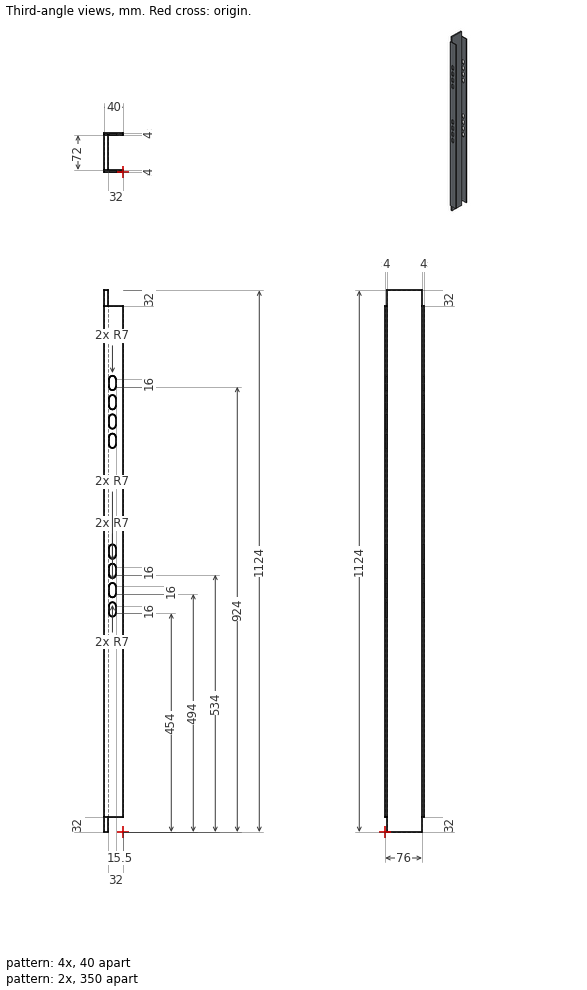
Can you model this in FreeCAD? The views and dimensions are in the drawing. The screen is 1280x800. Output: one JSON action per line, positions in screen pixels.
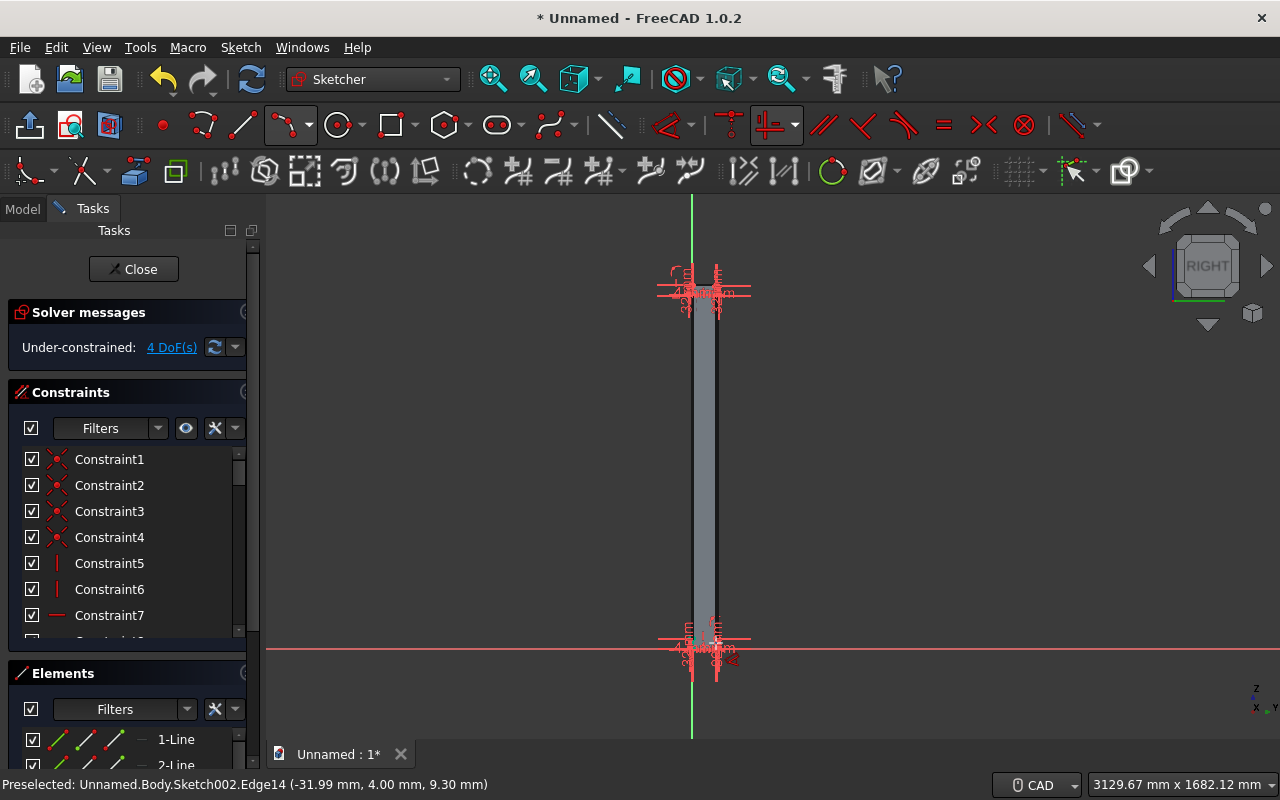
{"action": "scroll", "coordinate": [716, 286], "scroll_direction": "up", "scroll_amount": 12}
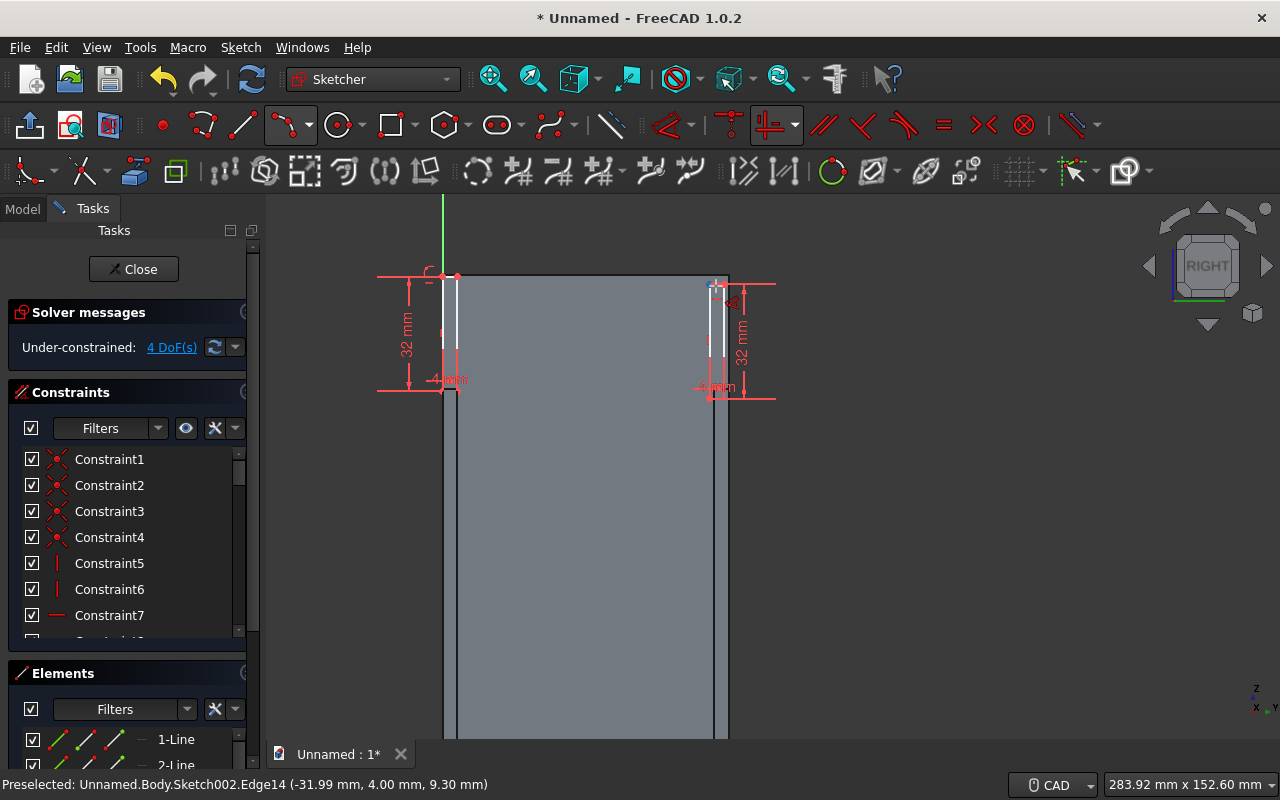
{"action": "left_click", "coordinate": [710, 284]}
{"action": "left_click", "coordinate": [576, 250]}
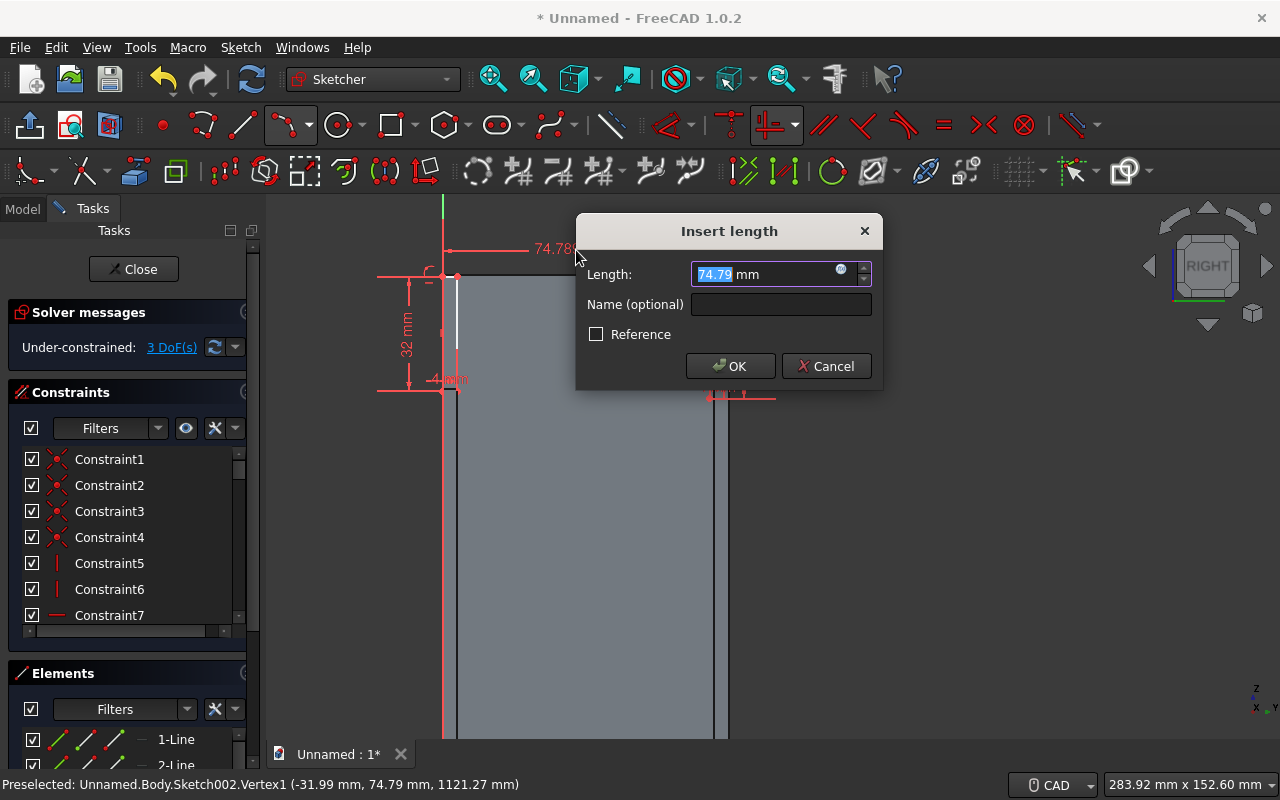
{"action": "type", "text": "76"}
{"action": "key", "text": "Return"}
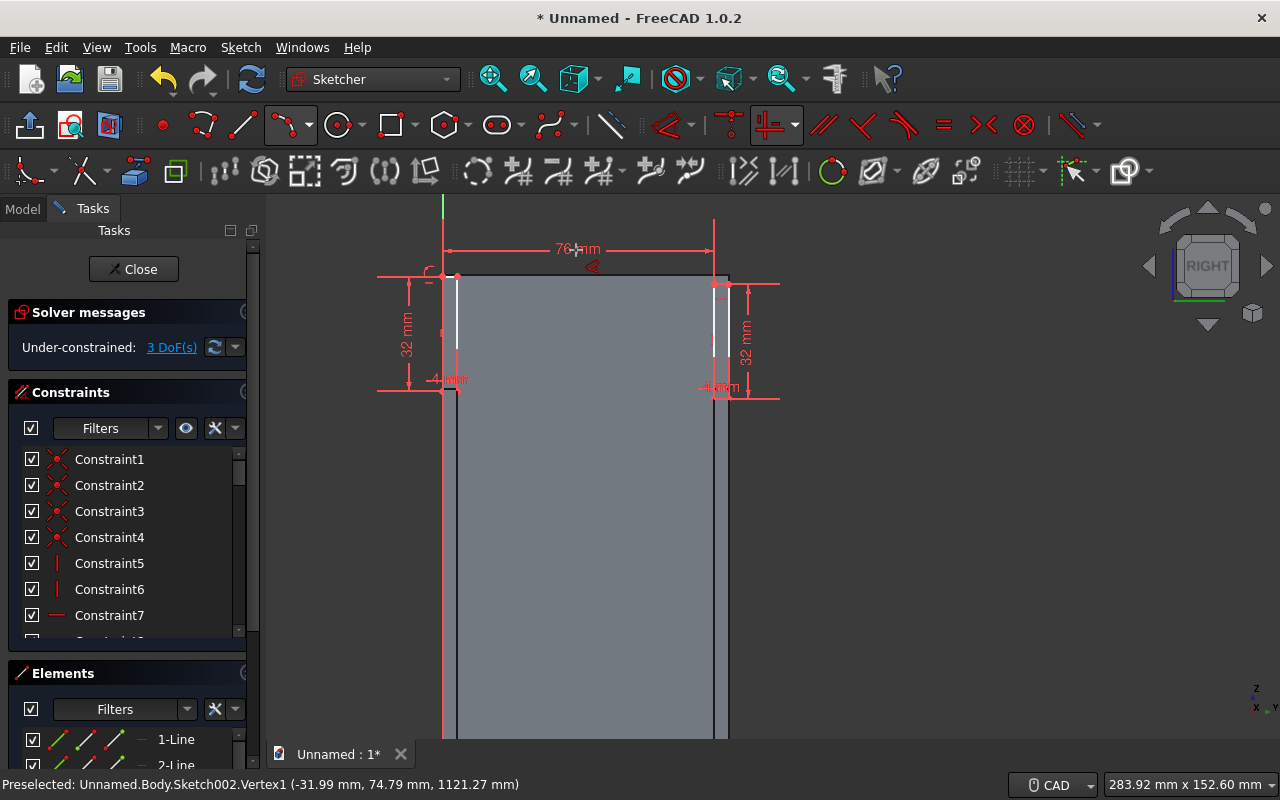
{"action": "scroll", "coordinate": [716, 285], "scroll_direction": "down", "scroll_amount": 12}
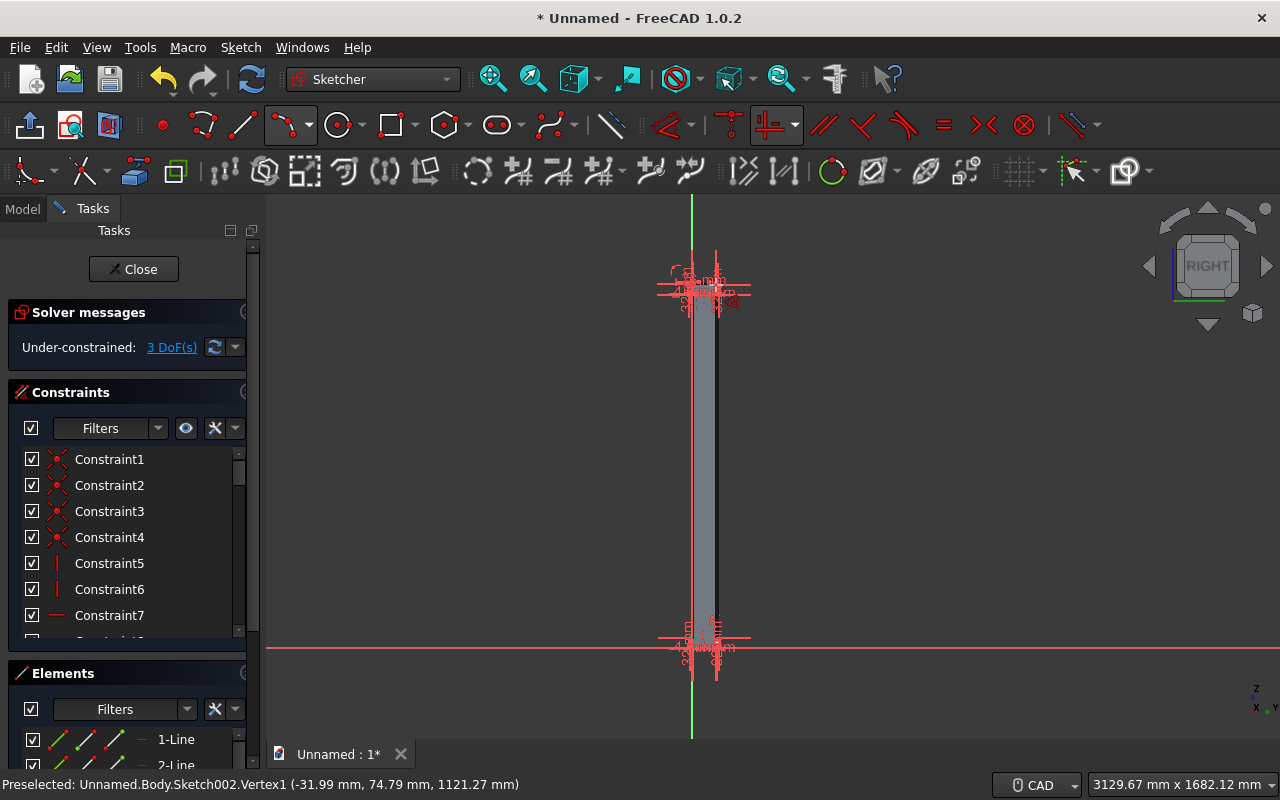
{"action": "scroll", "coordinate": [716, 638], "scroll_direction": "up", "scroll_amount": 12}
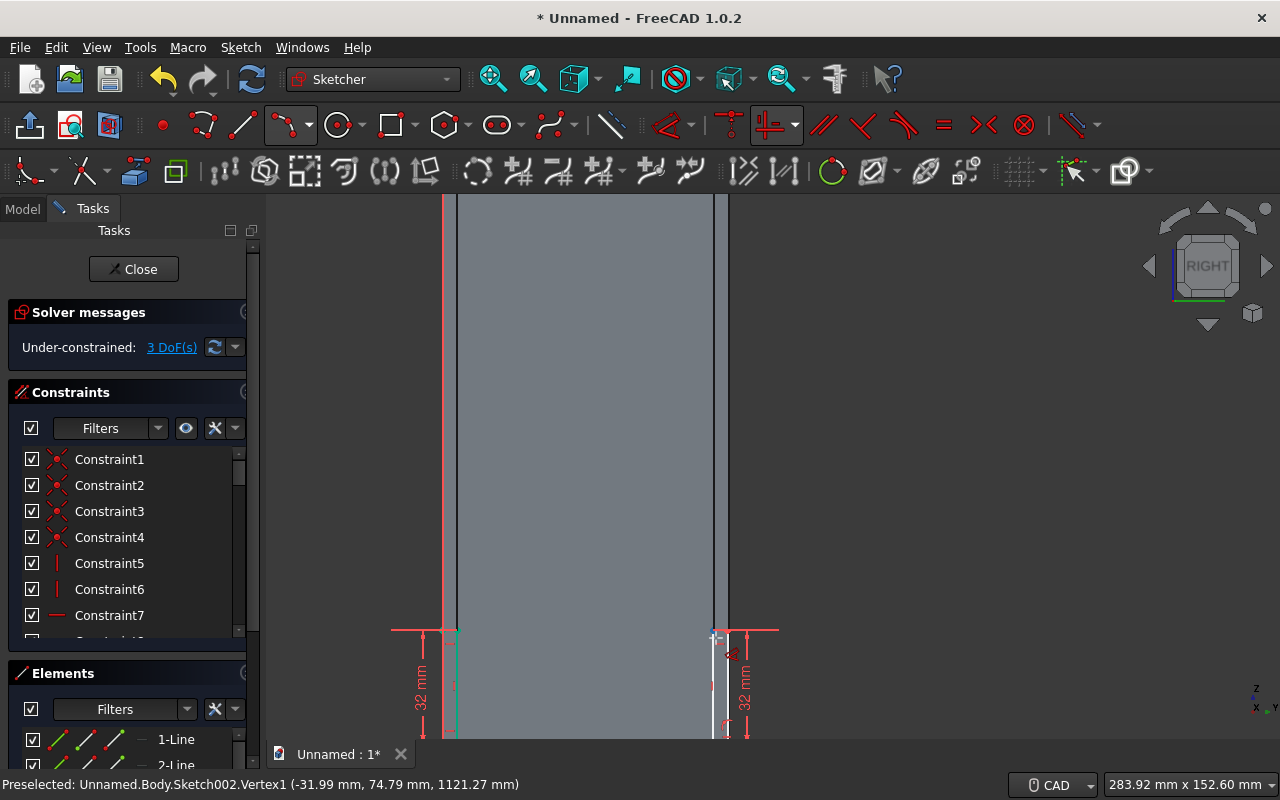
{"action": "left_click", "coordinate": [713, 630]}
{"action": "left_click", "coordinate": [578, 596]}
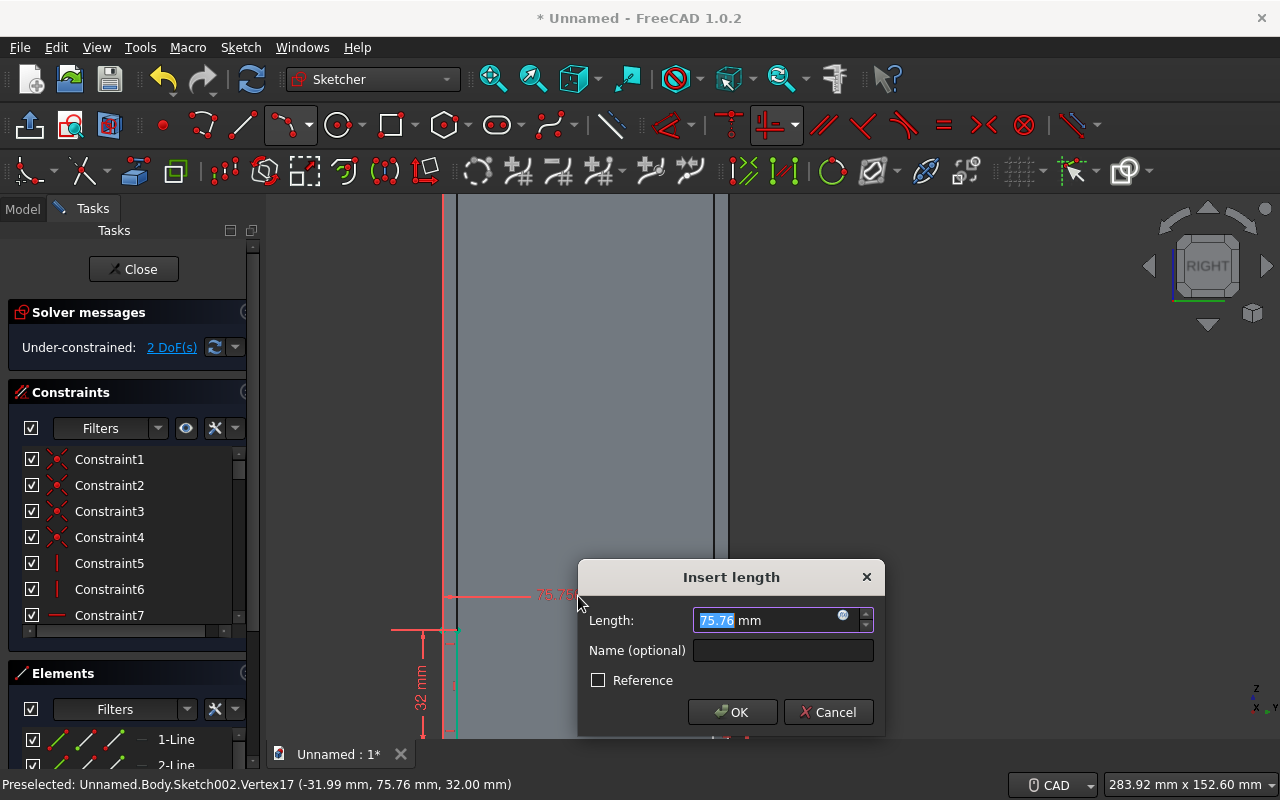
{"action": "type", "text": "76"}
{"action": "key", "text": "Return"}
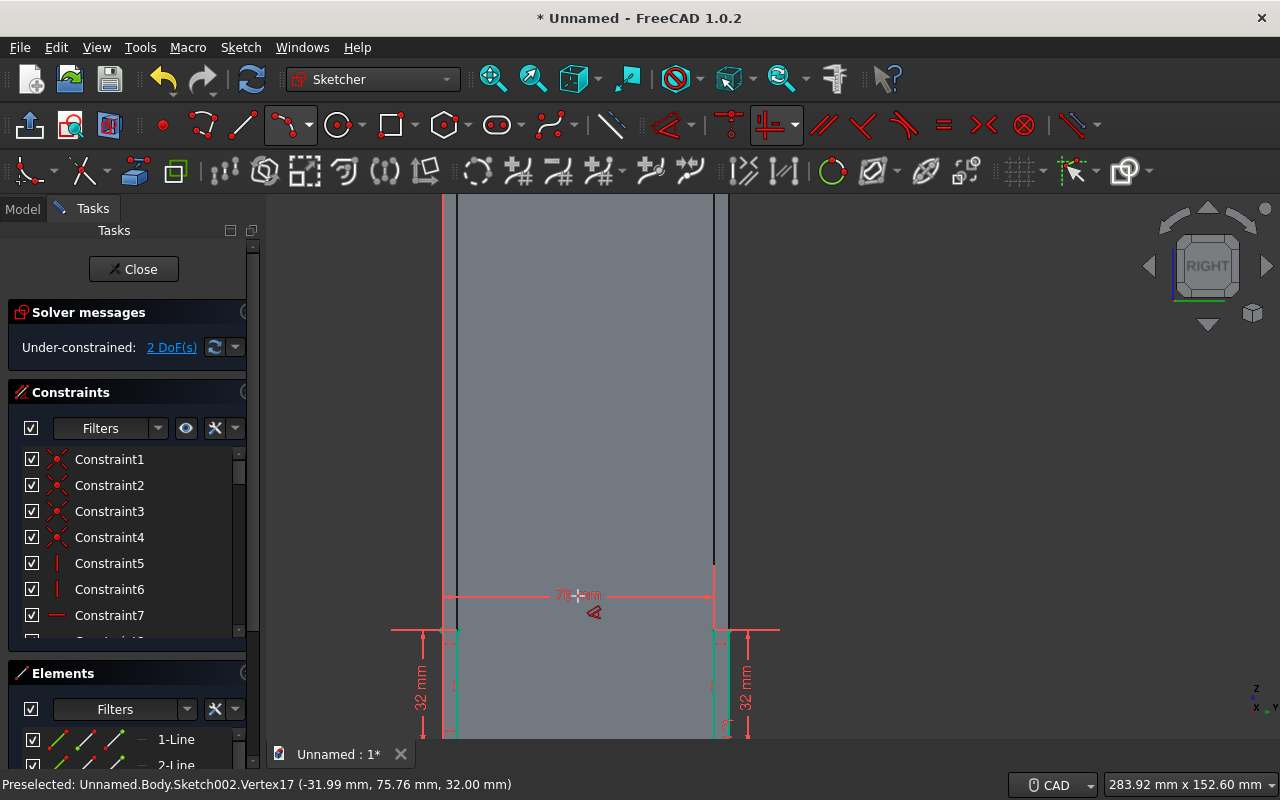
{"action": "scroll", "coordinate": [716, 639], "scroll_direction": "down", "scroll_amount": 12}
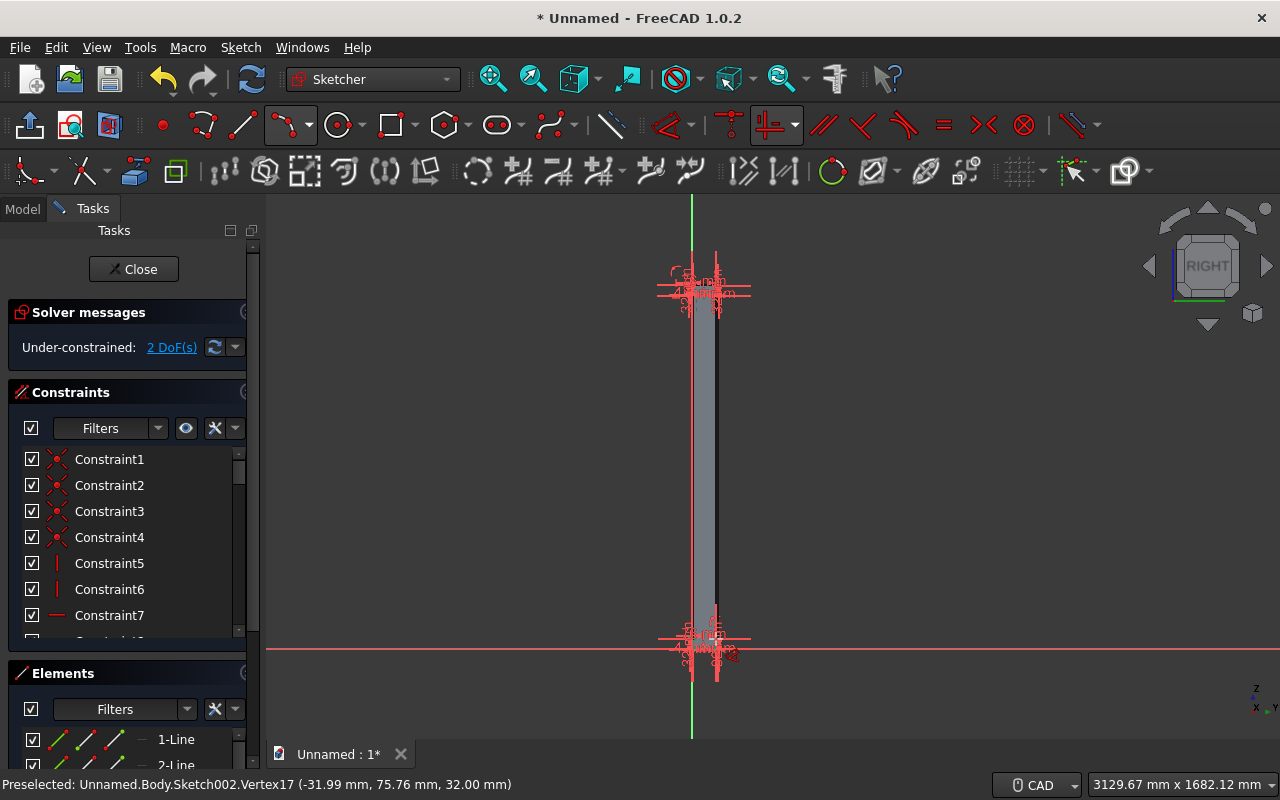
{"action": "scroll", "coordinate": [716, 286], "scroll_direction": "up", "scroll_amount": 12}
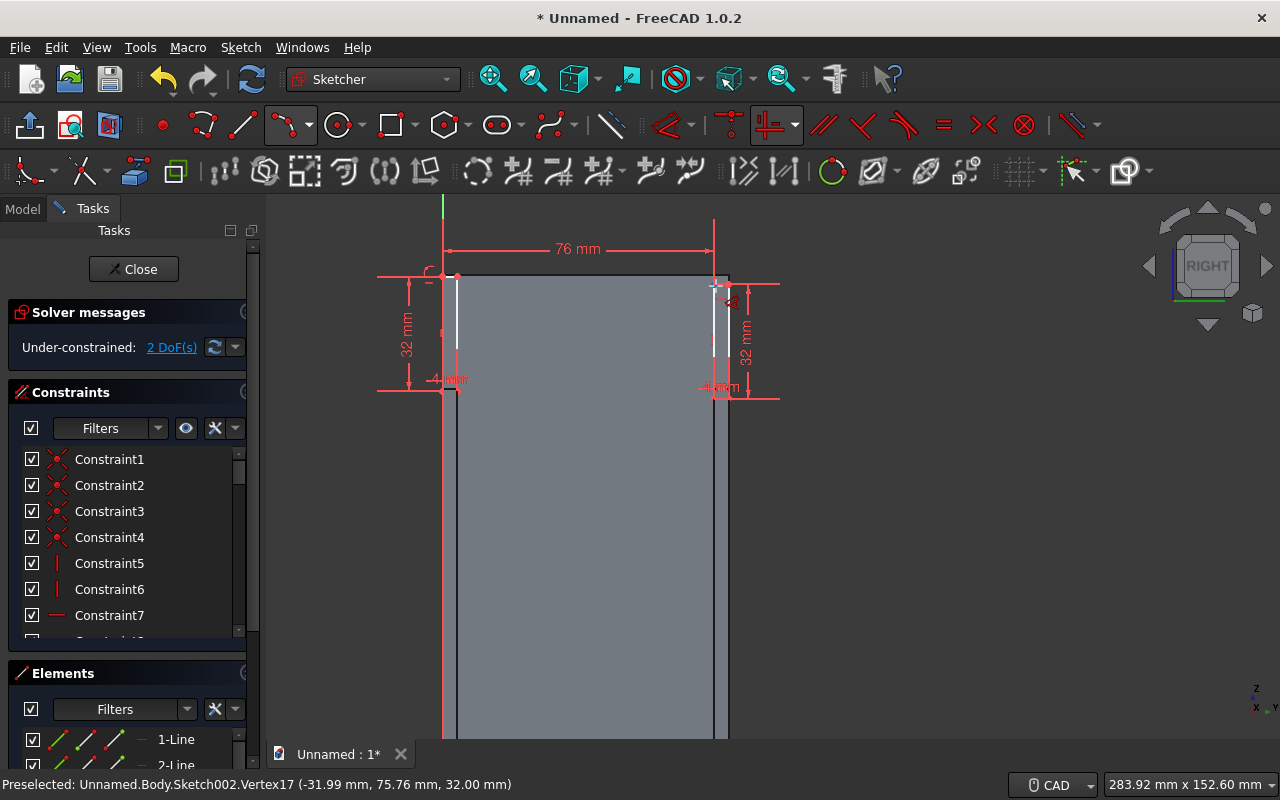
{"action": "left_click", "coordinate": [714, 284]}
{"action": "left_click", "coordinate": [409, 498]}